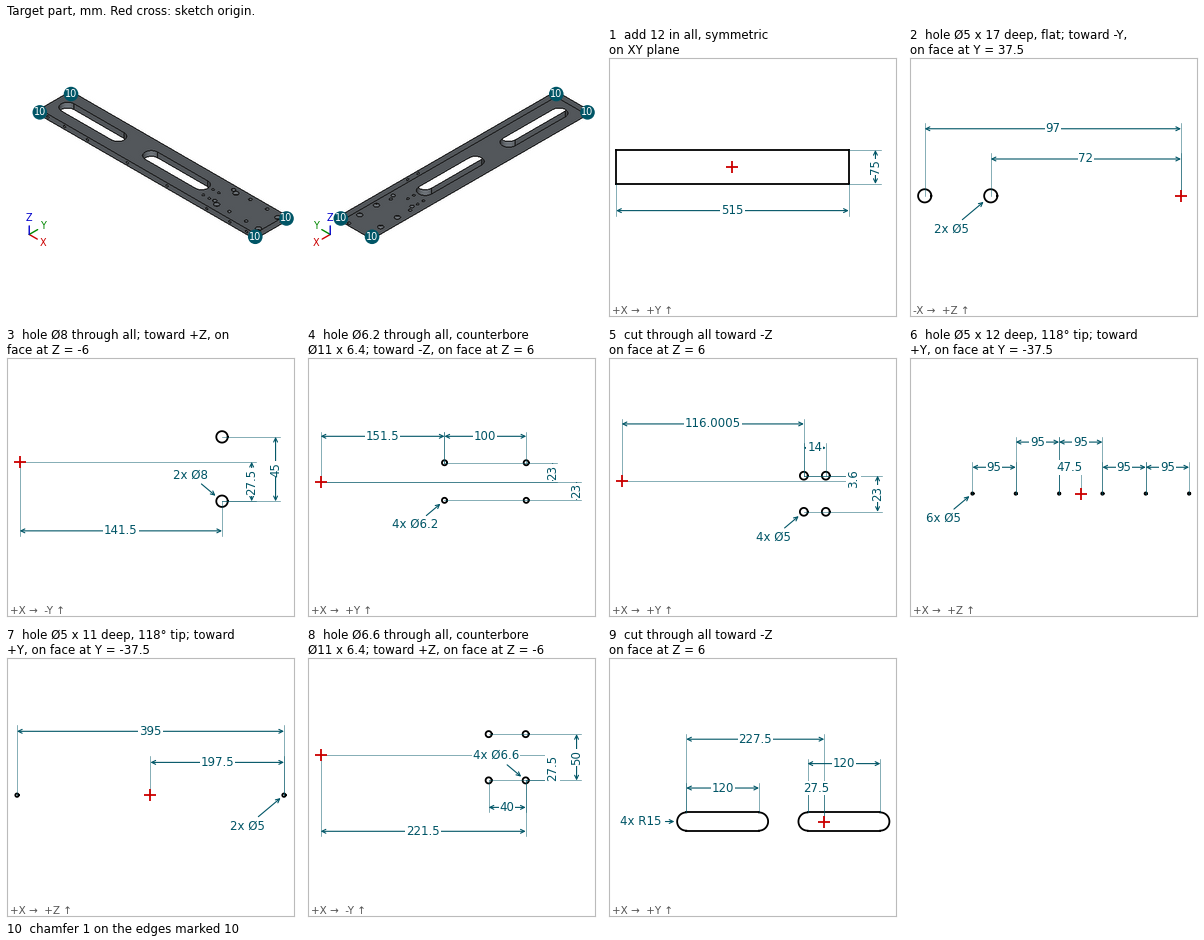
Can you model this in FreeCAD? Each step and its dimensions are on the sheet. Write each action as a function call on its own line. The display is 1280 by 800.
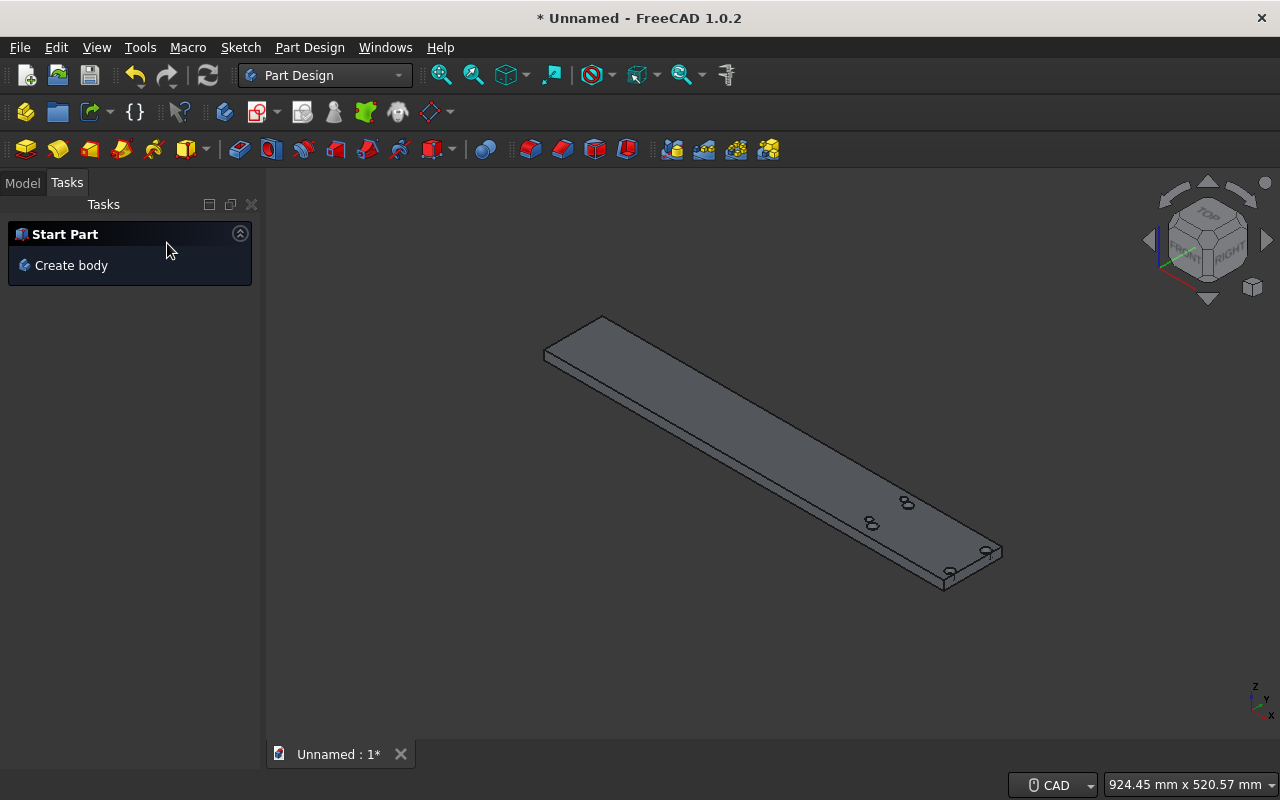
click(830, 480)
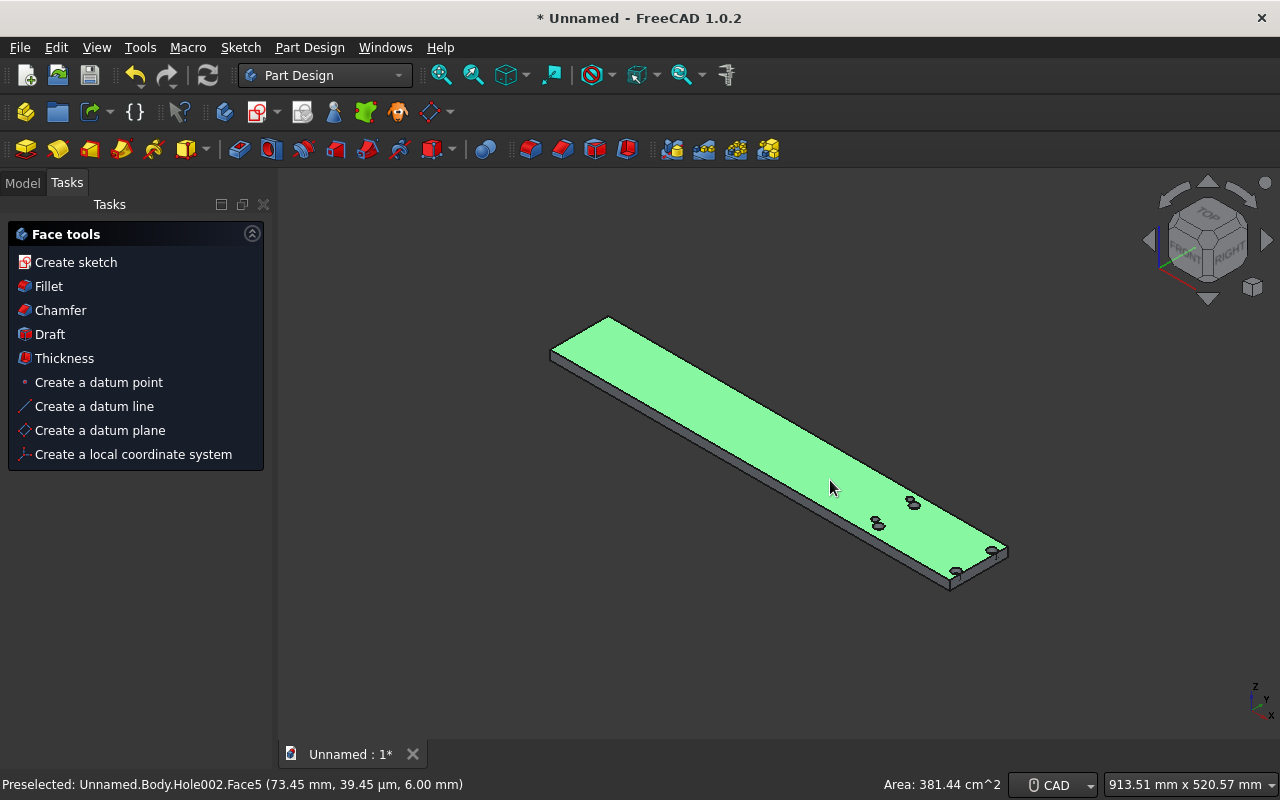
click(258, 112)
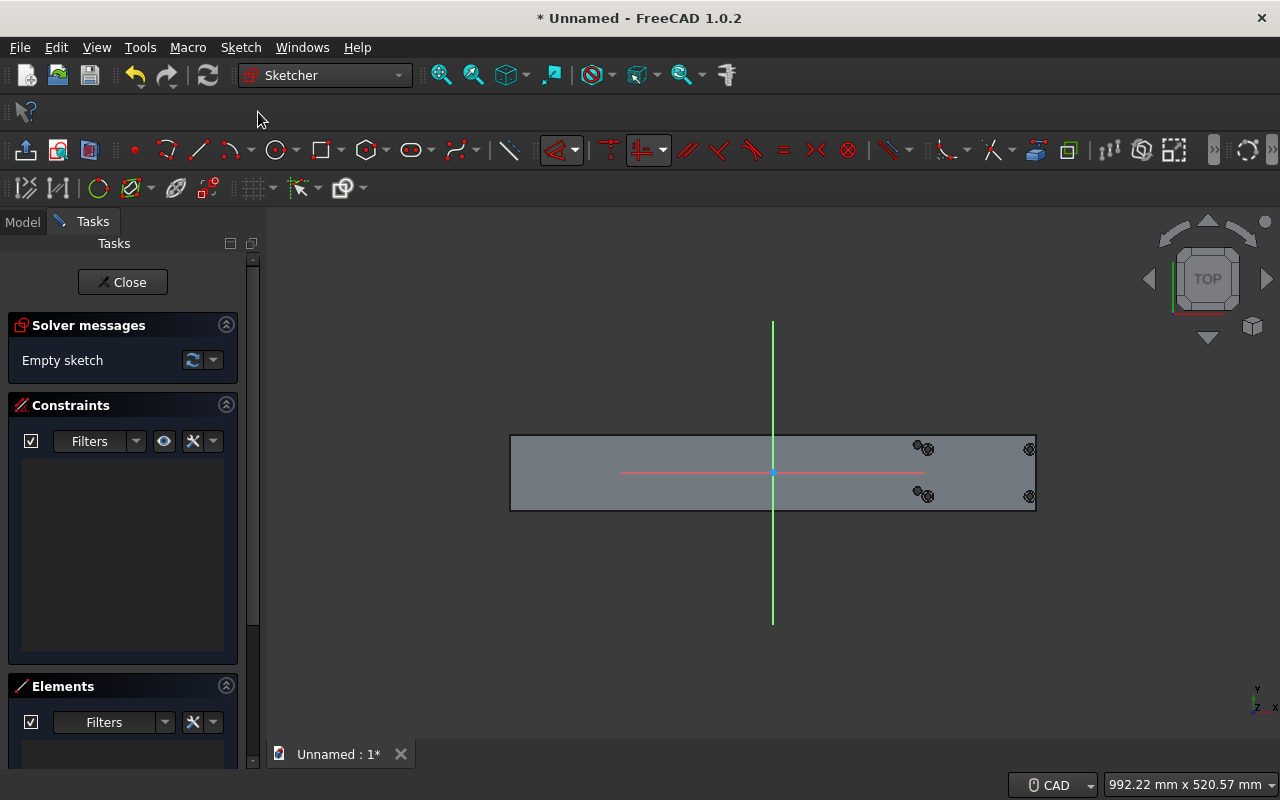
scroll(918, 482, up, 12)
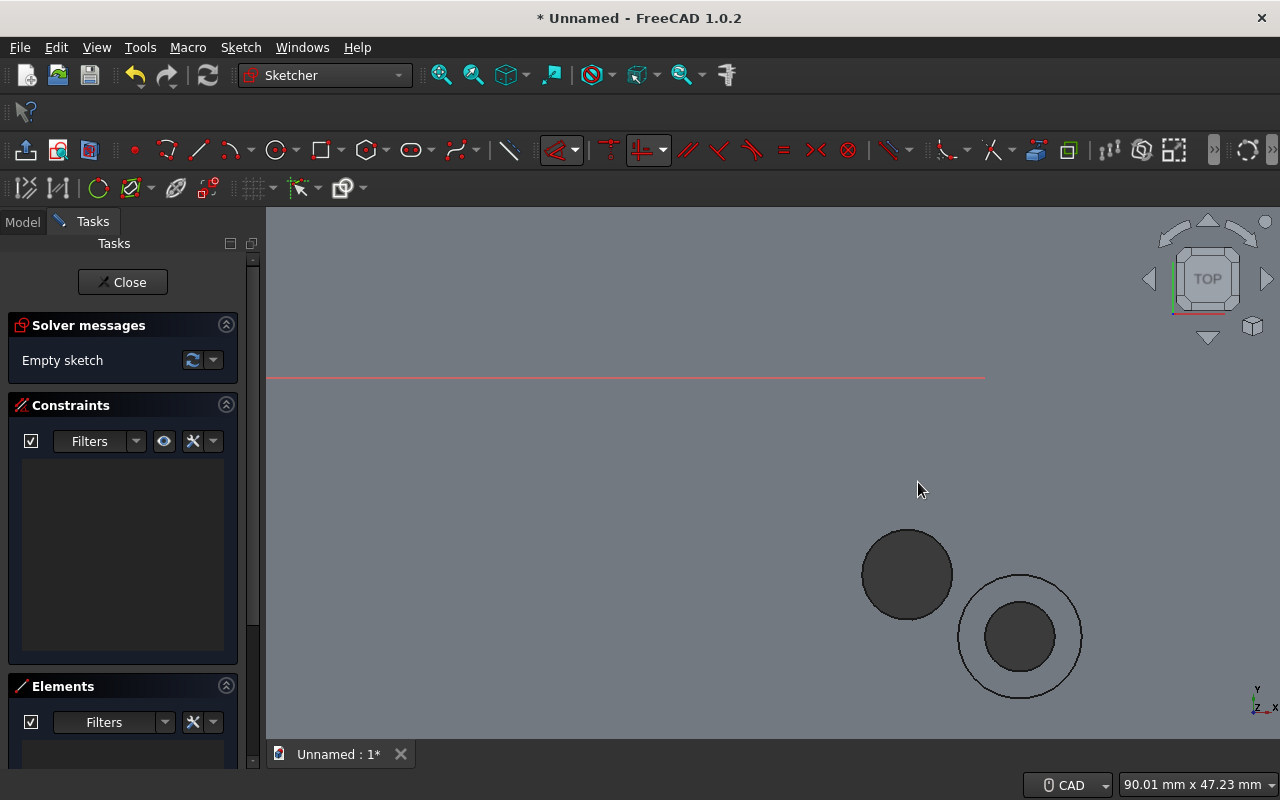
key(g)
key(c)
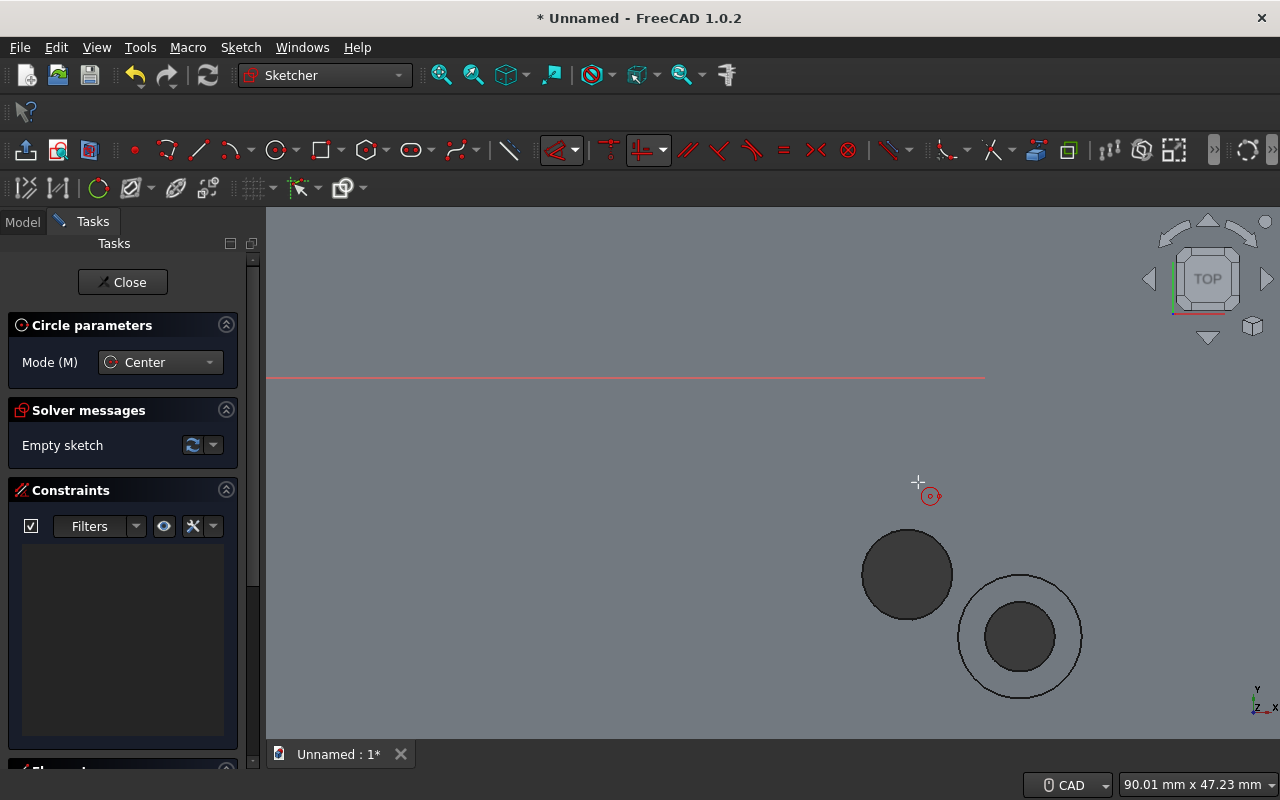
click(620, 337)
click(640, 317)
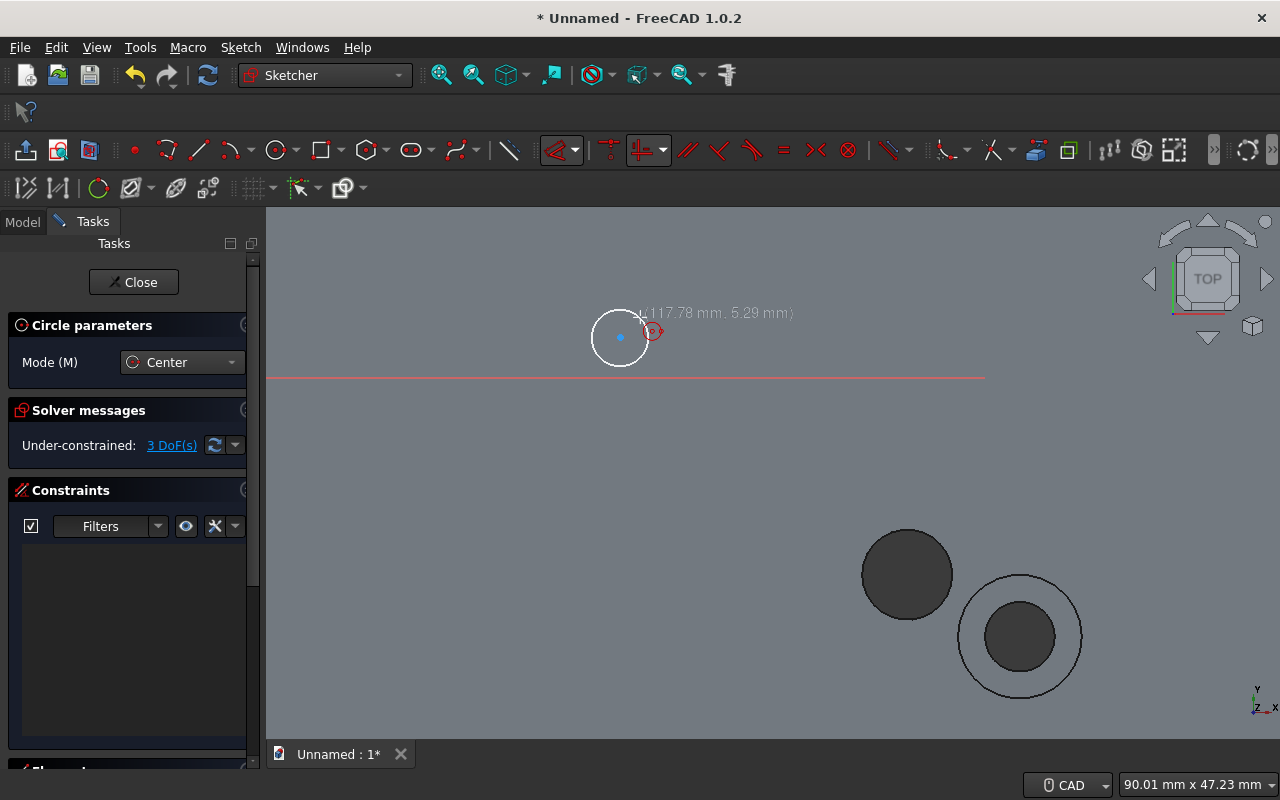
click(778, 337)
click(798, 317)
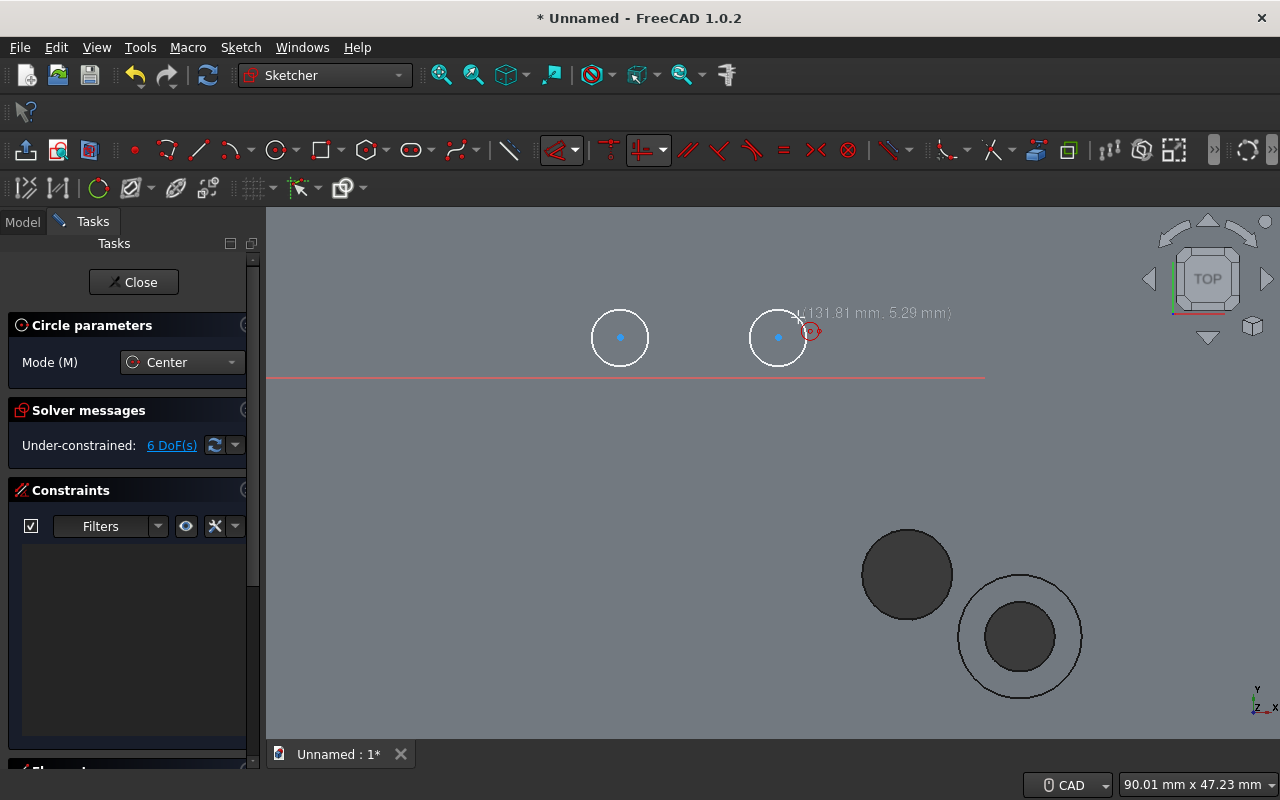
click(620, 596)
click(640, 576)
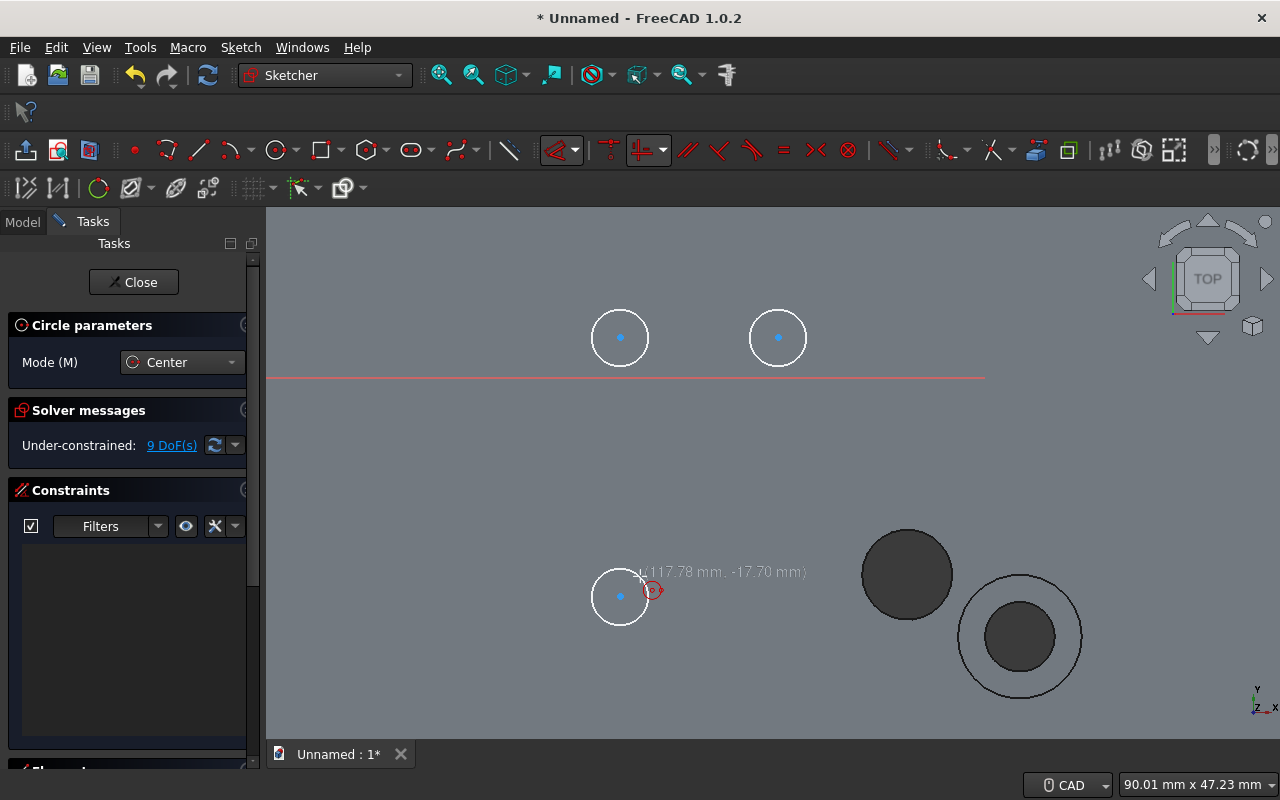
click(778, 596)
click(798, 576)
key(Escape)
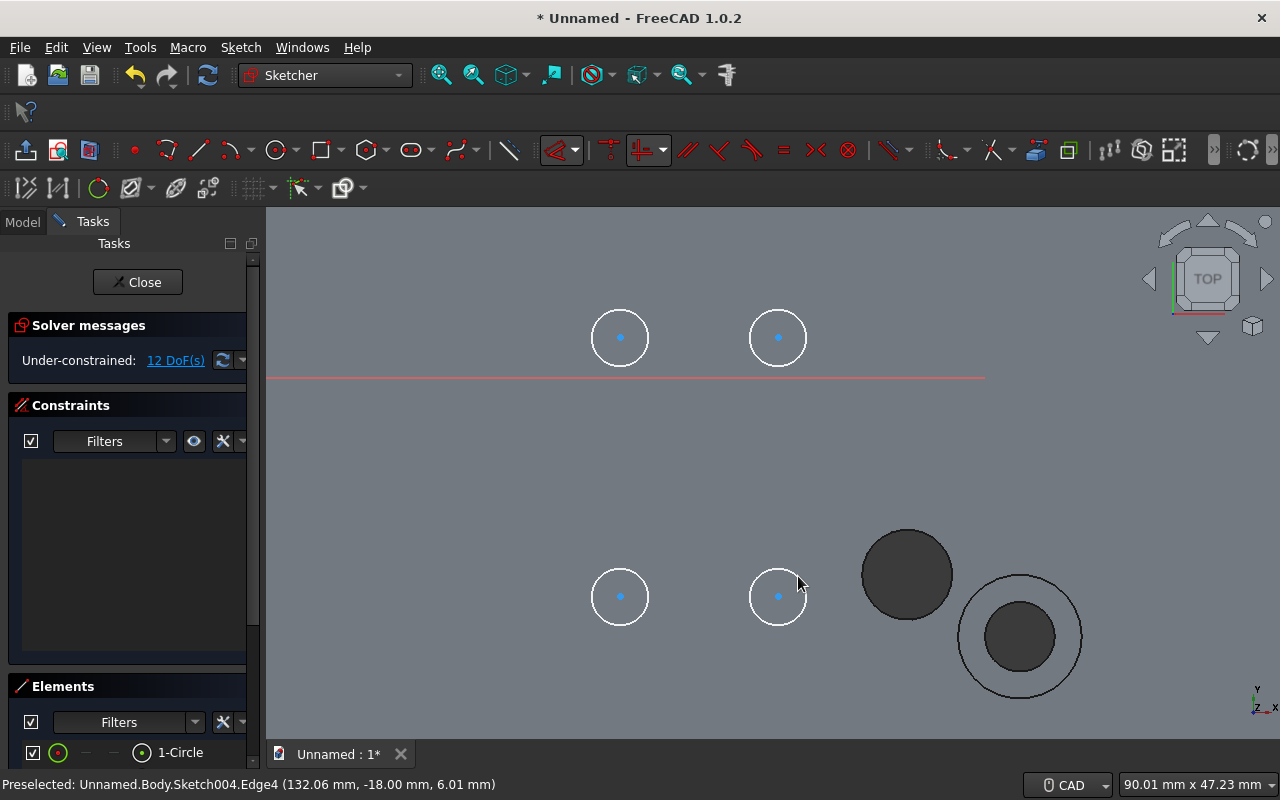
click(640, 318)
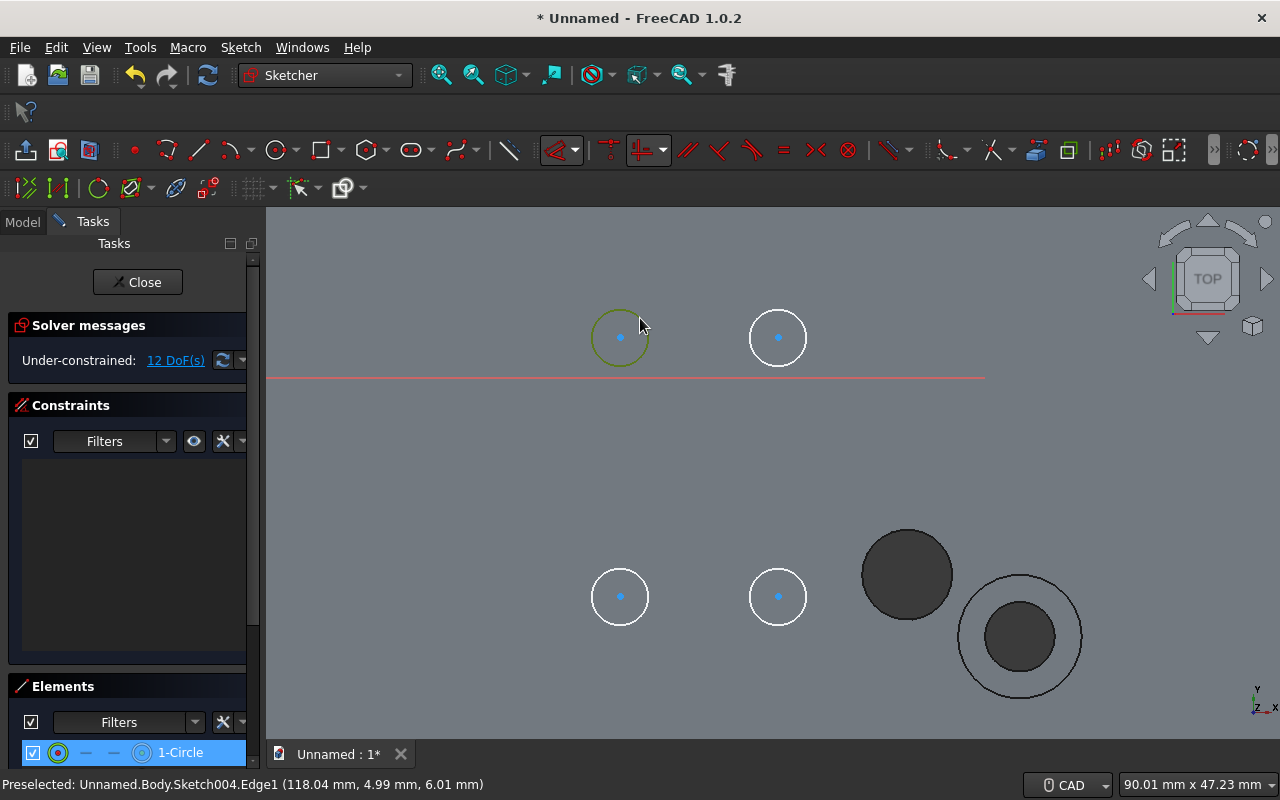
click(798, 318)